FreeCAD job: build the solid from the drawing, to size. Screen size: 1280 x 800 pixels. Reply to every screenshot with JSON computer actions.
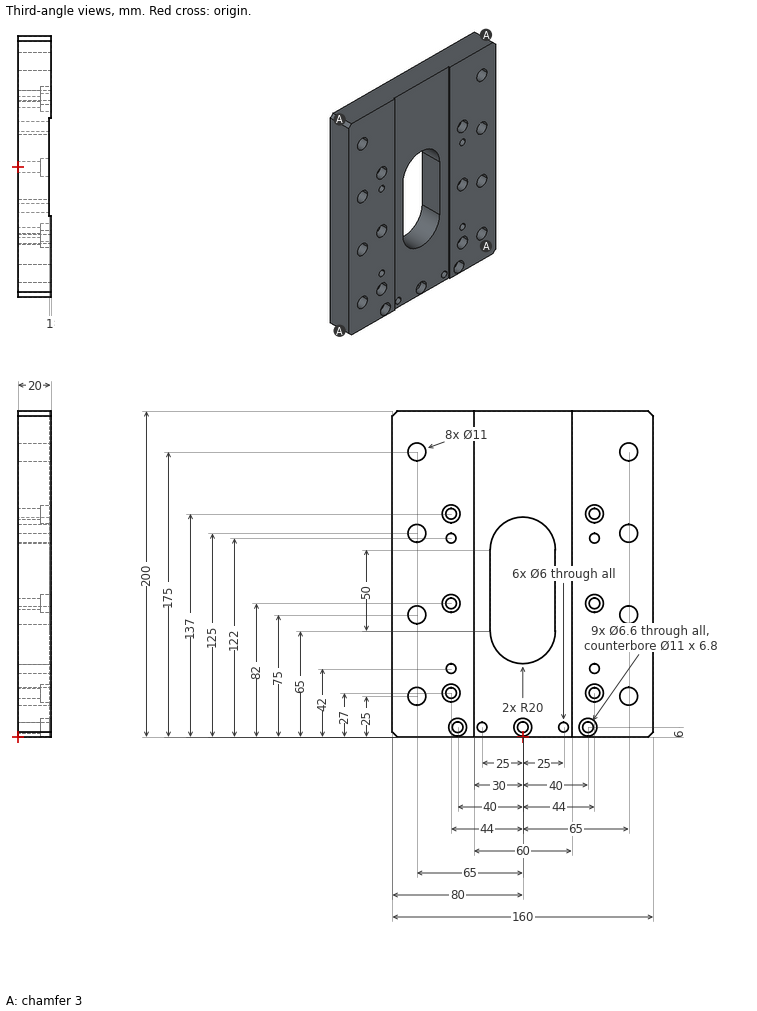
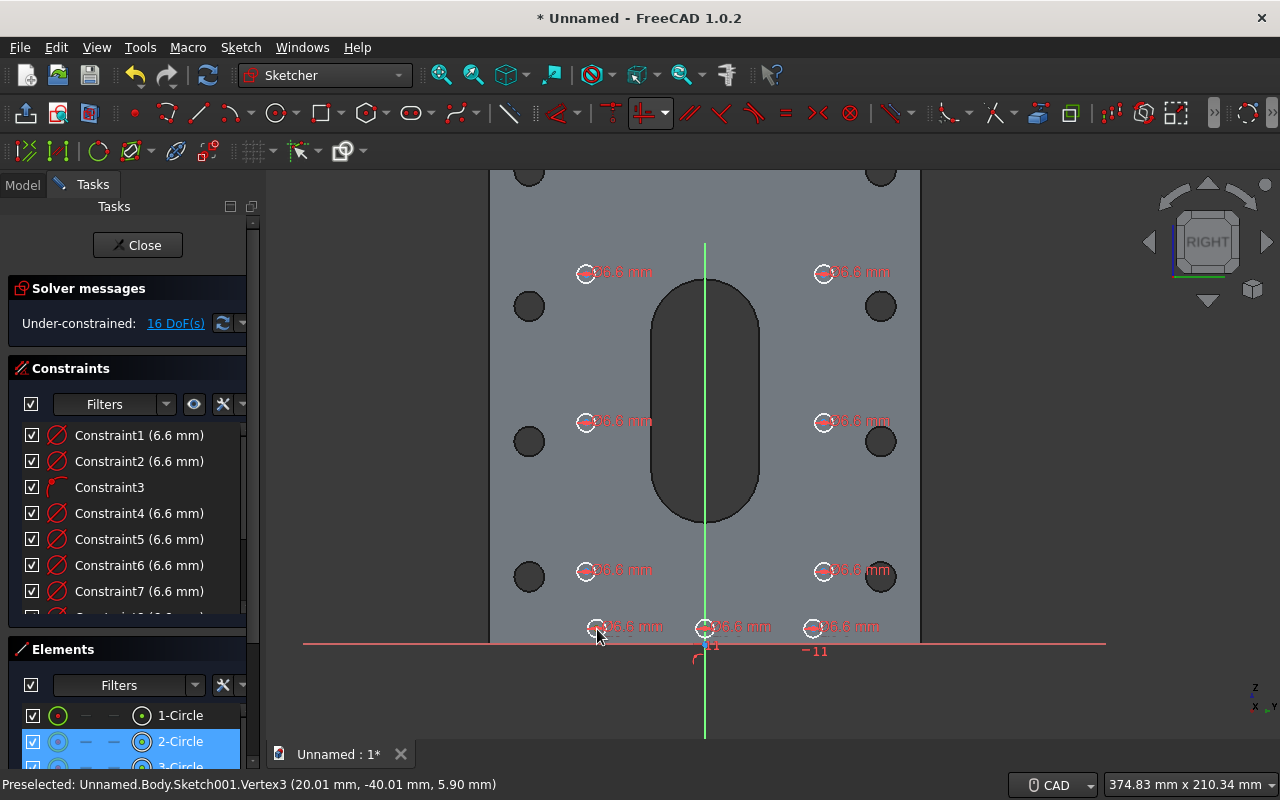
{"action": "key", "text": "h"}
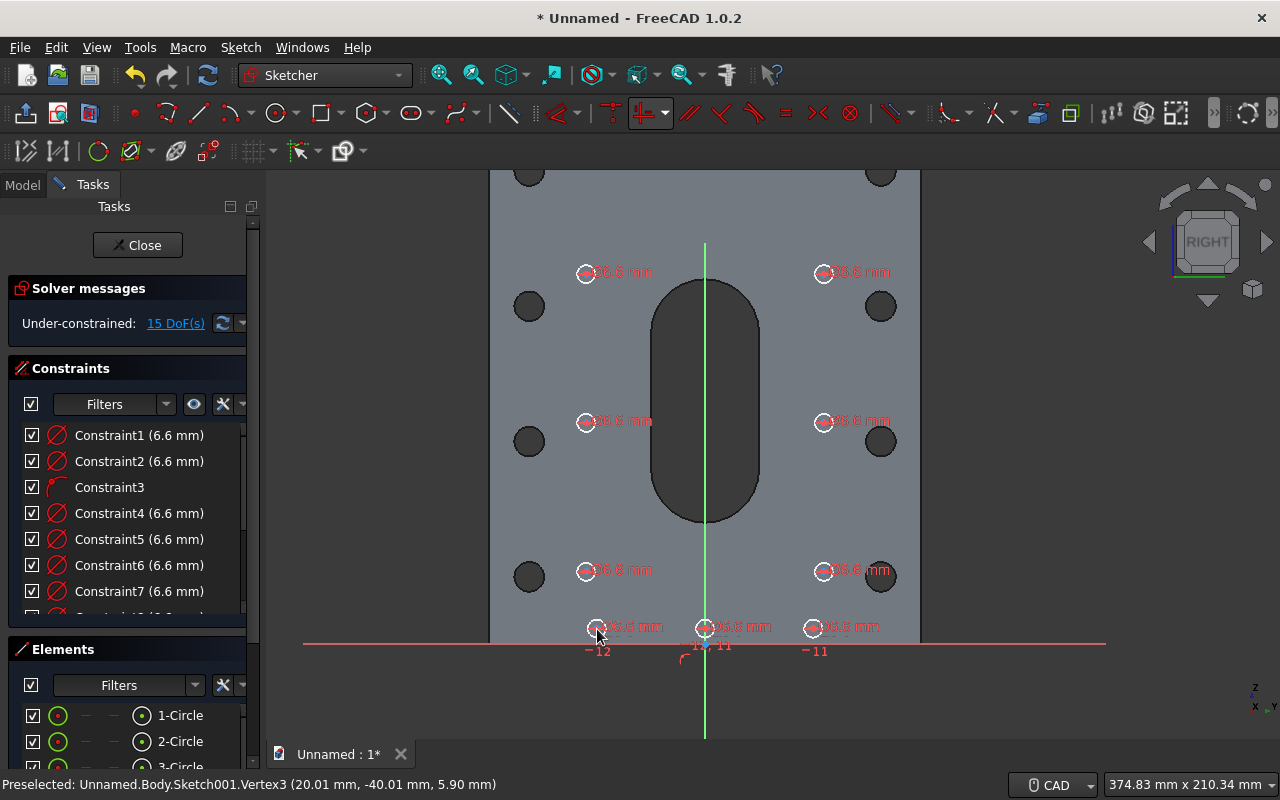
{"action": "left_click", "coordinate": [586, 572]}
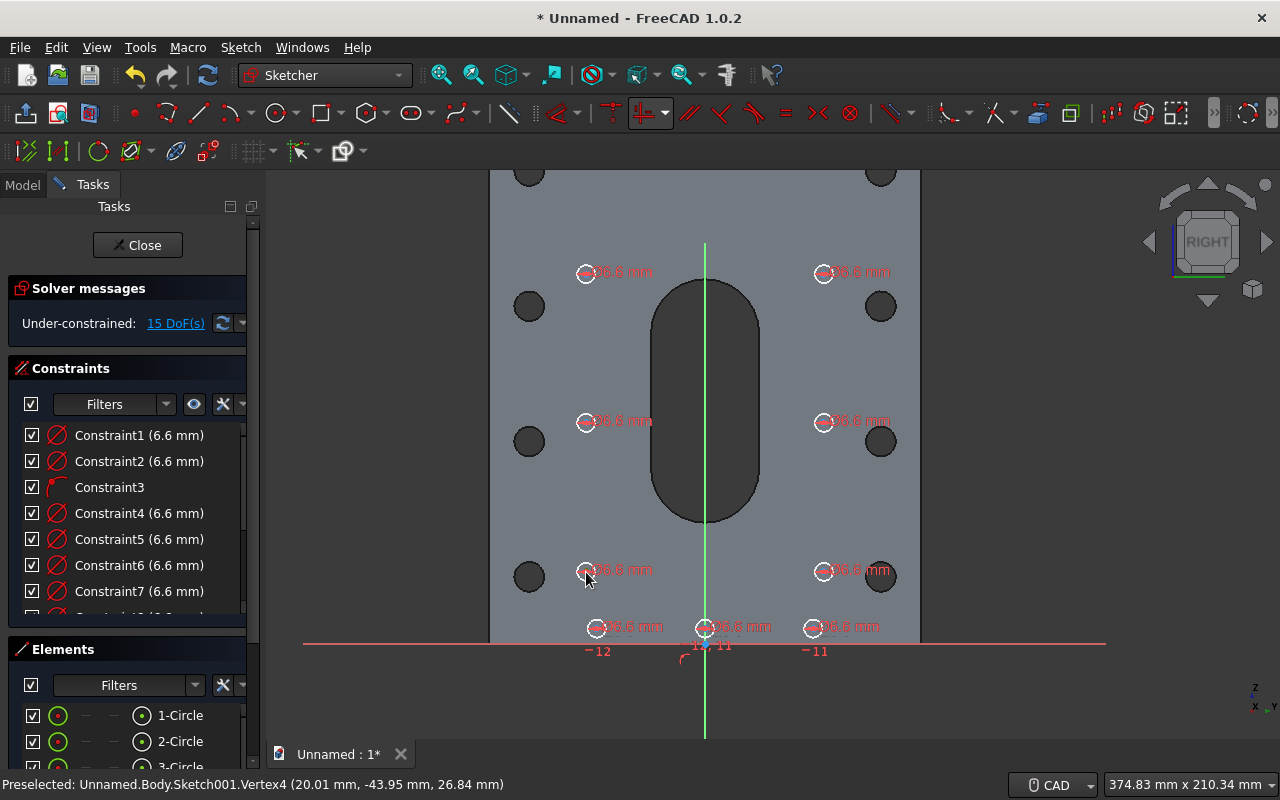
{"action": "left_click", "coordinate": [586, 423]}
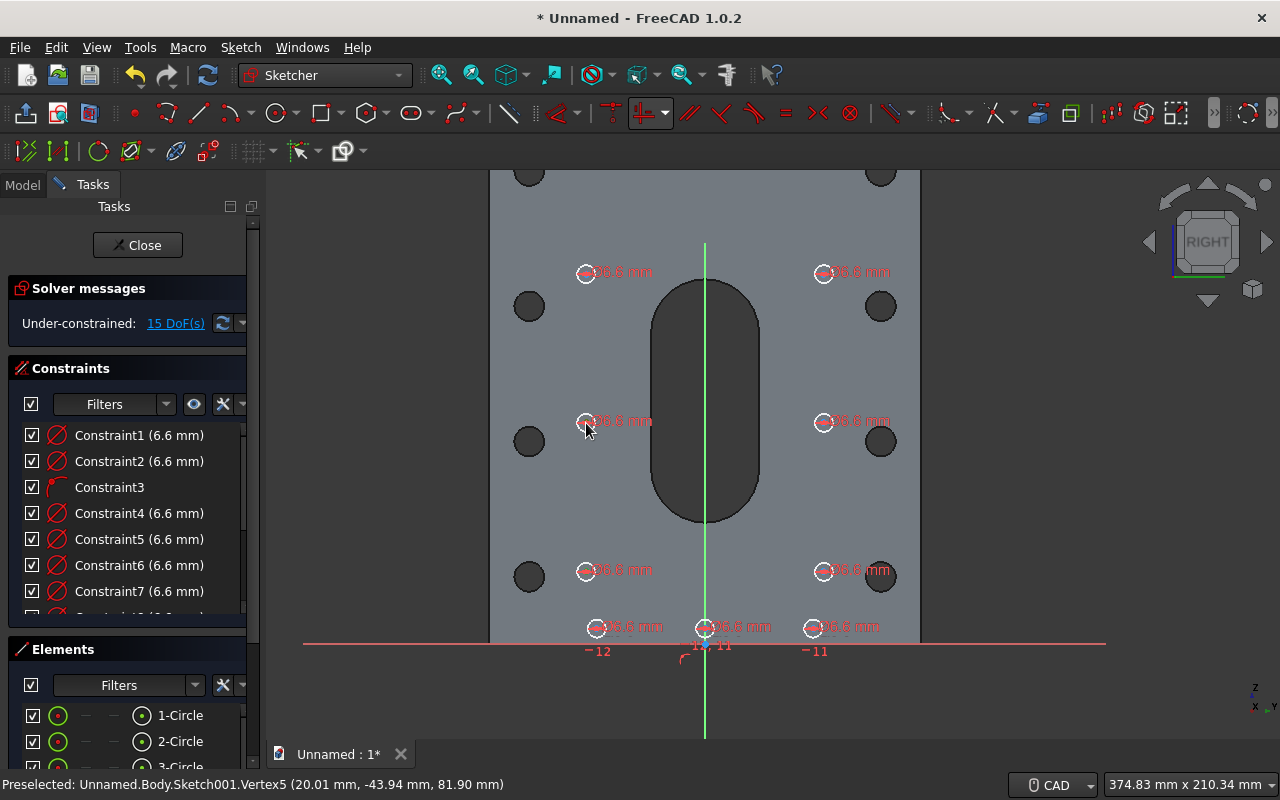
{"action": "key", "text": "v"}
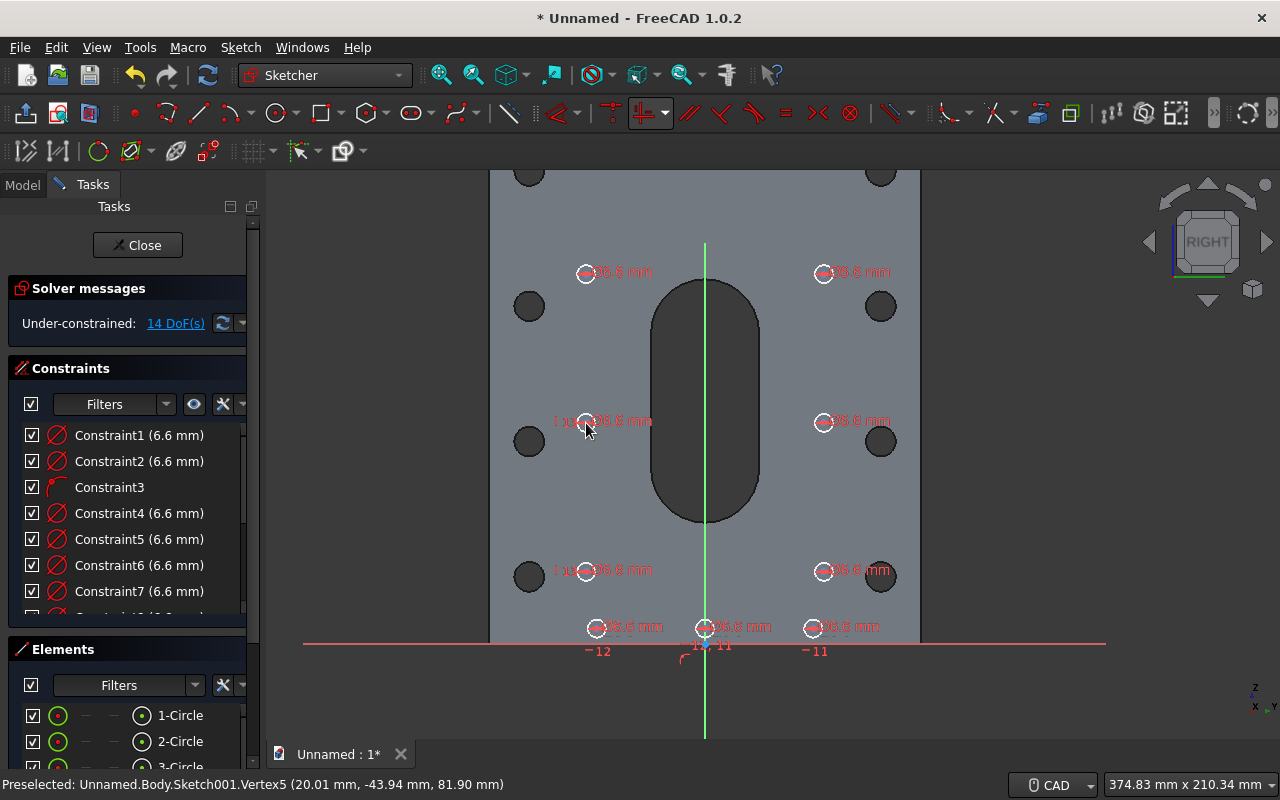
{"action": "left_click", "coordinate": [586, 423]}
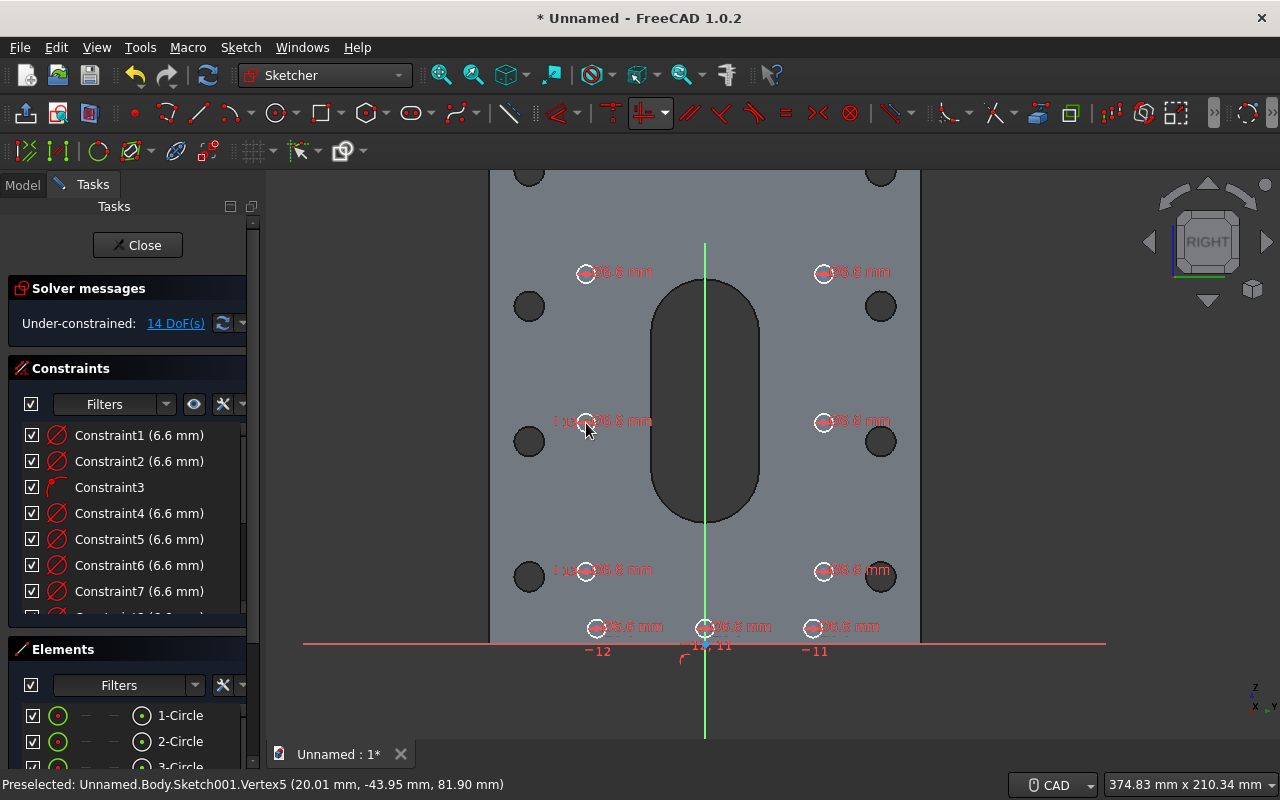
{"action": "left_click", "coordinate": [586, 274]}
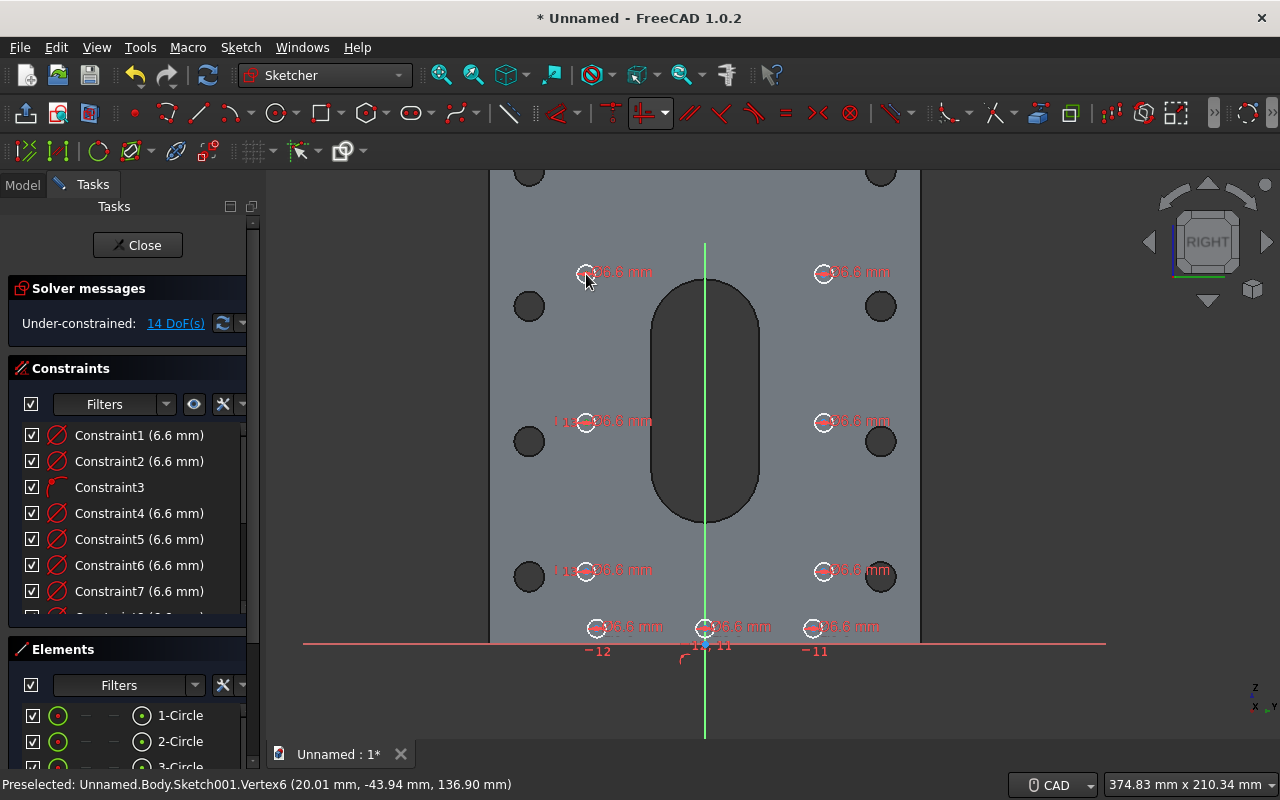
{"action": "key", "text": "v"}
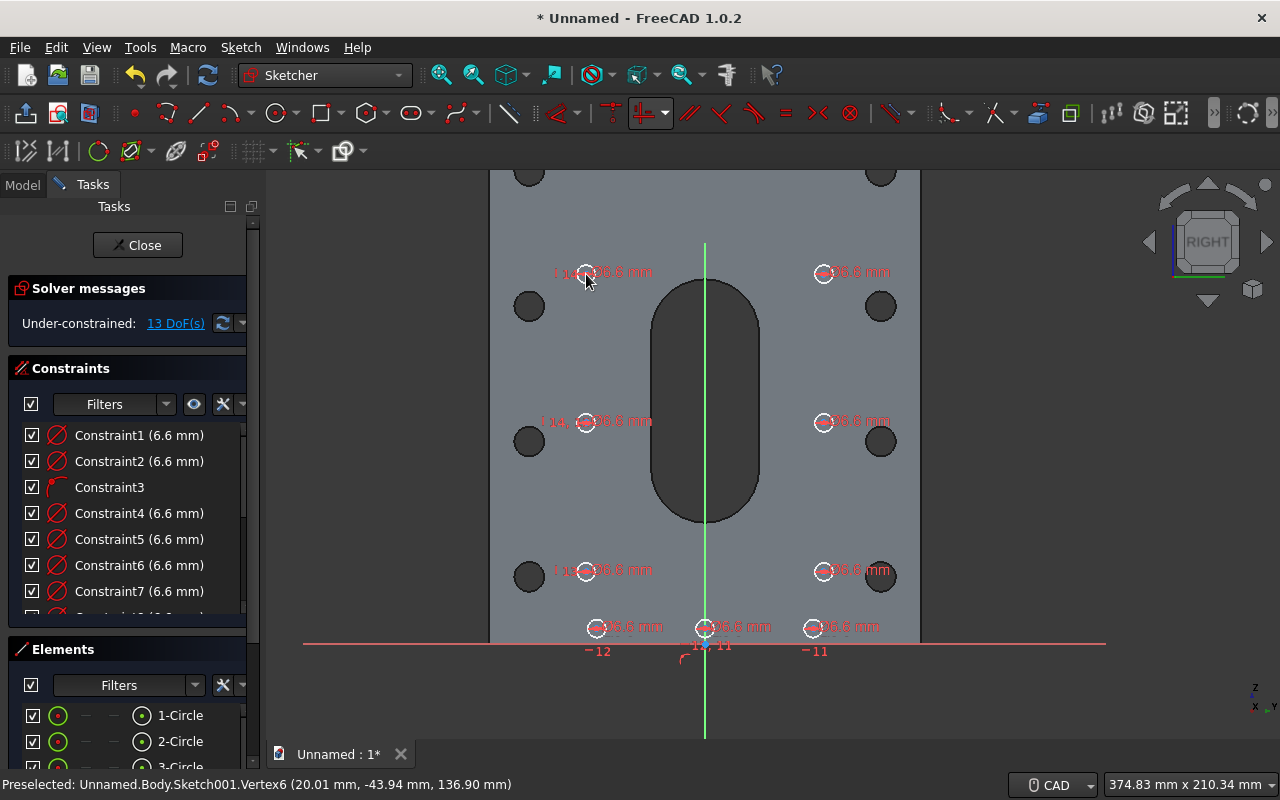
{"action": "left_click", "coordinate": [586, 572]}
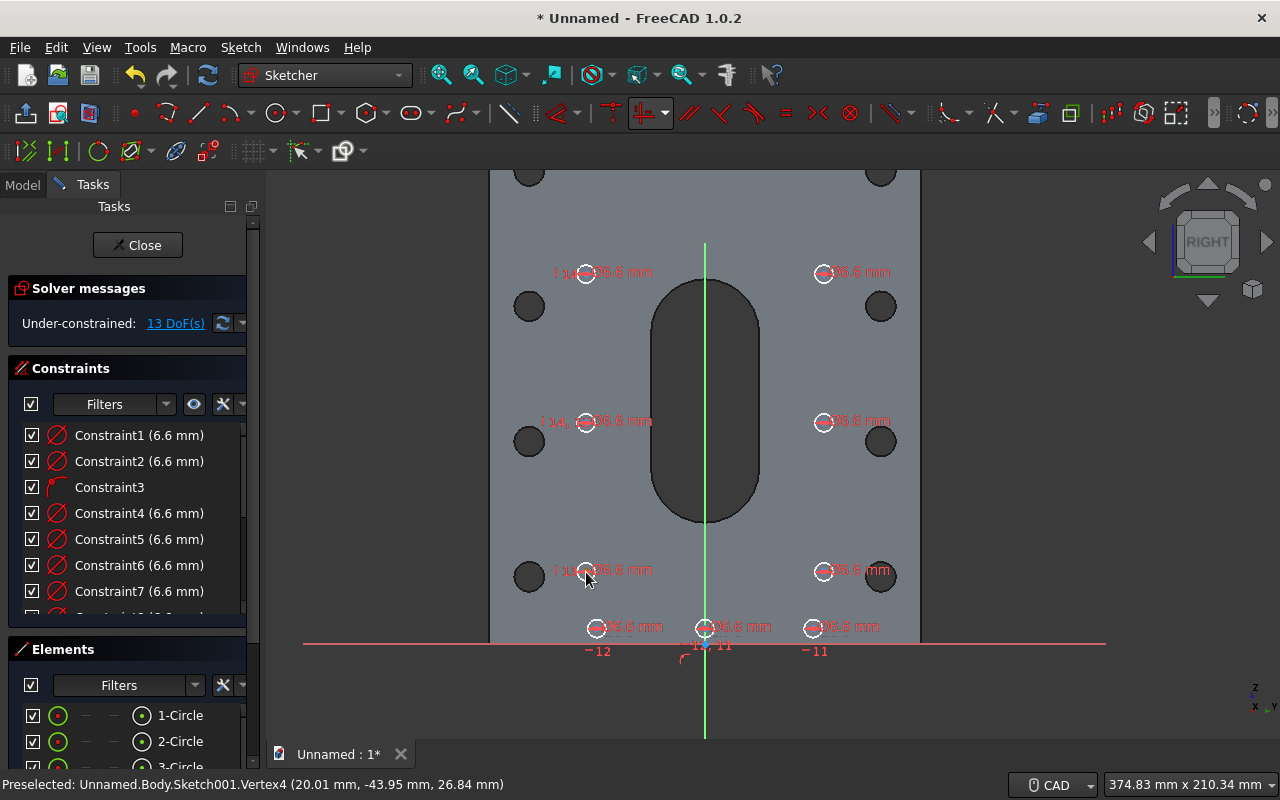
{"action": "left_click", "coordinate": [824, 572]}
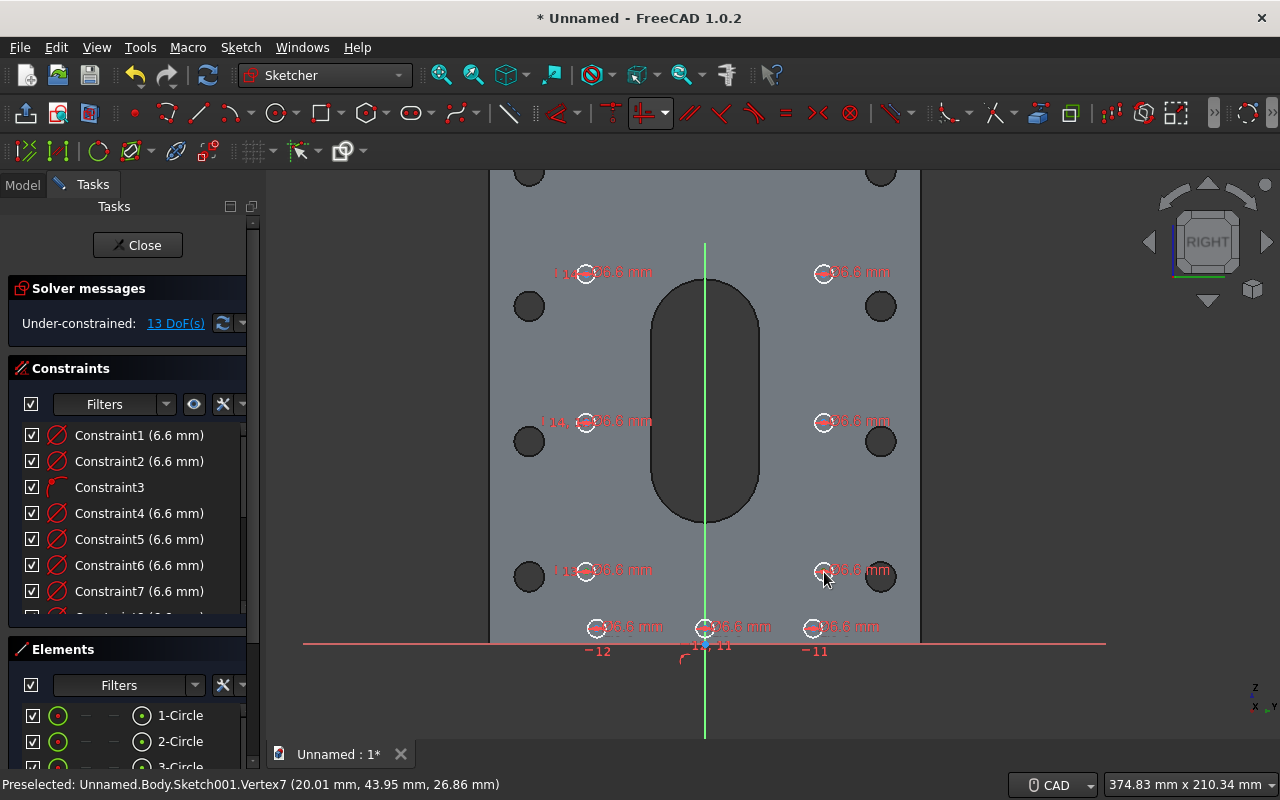
{"action": "key", "text": "h"}